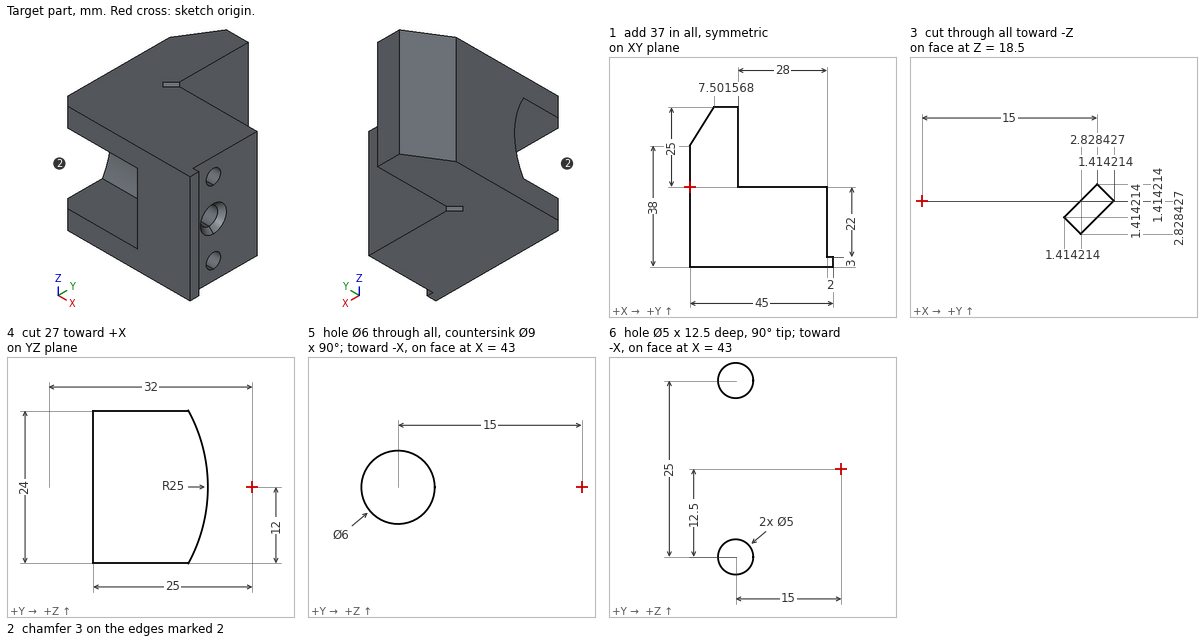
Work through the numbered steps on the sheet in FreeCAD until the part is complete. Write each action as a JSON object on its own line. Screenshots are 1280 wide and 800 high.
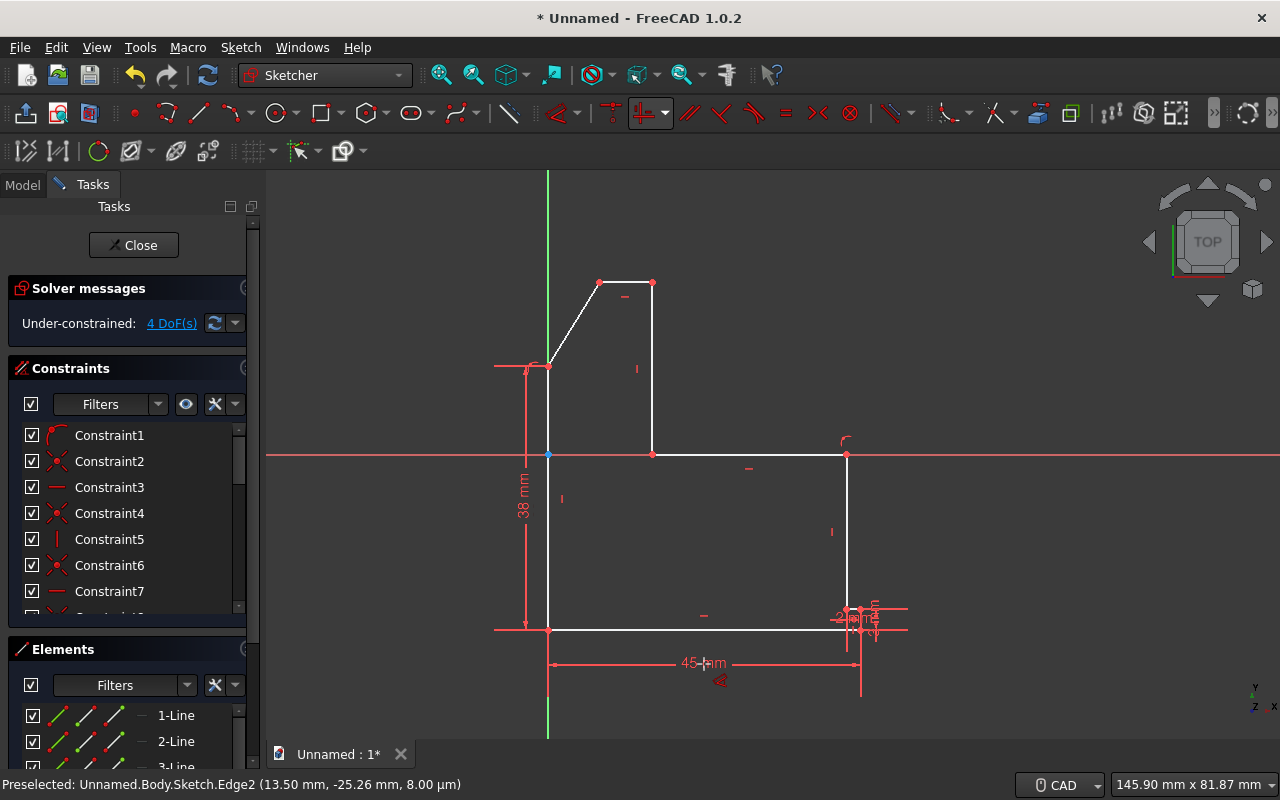
{"action": "left_click", "coordinate": [847, 563]}
{"action": "left_click", "coordinate": [881, 532]}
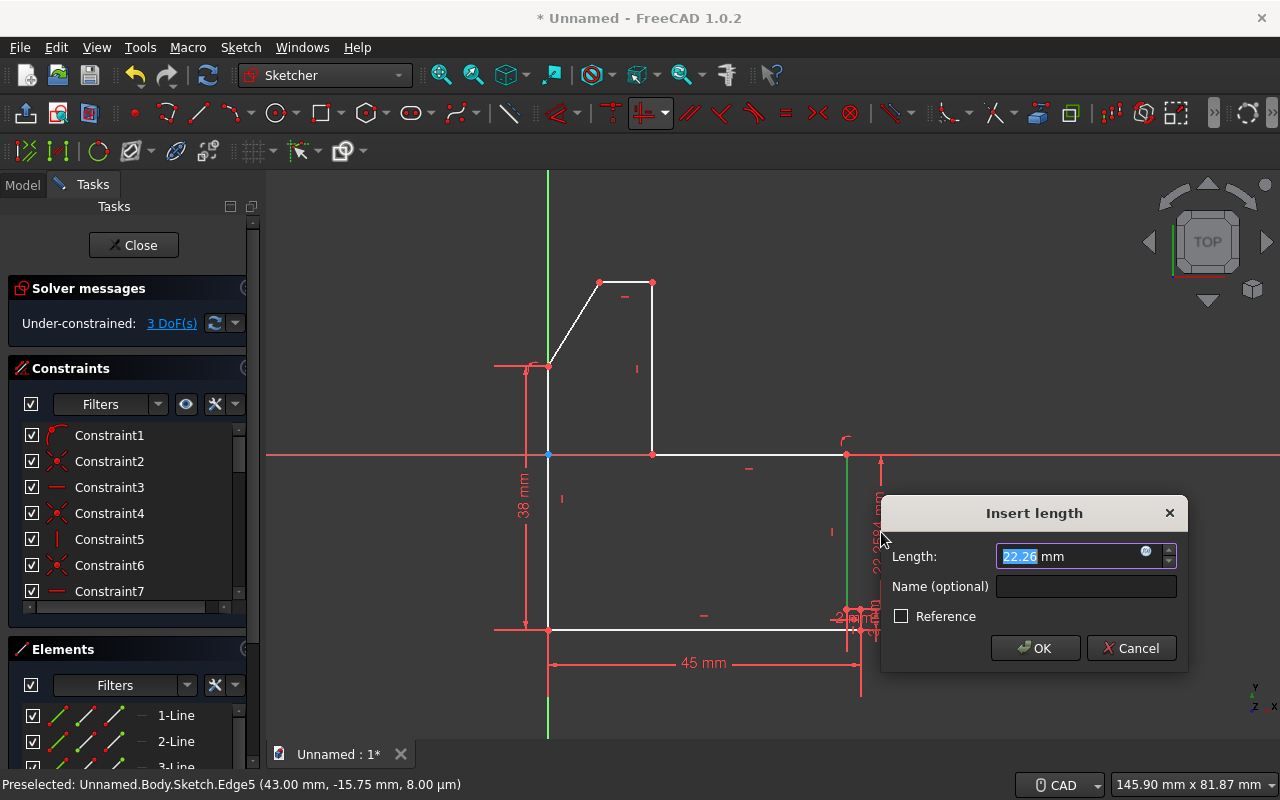
{"action": "type", "text": "22"}
{"action": "key", "text": "Return"}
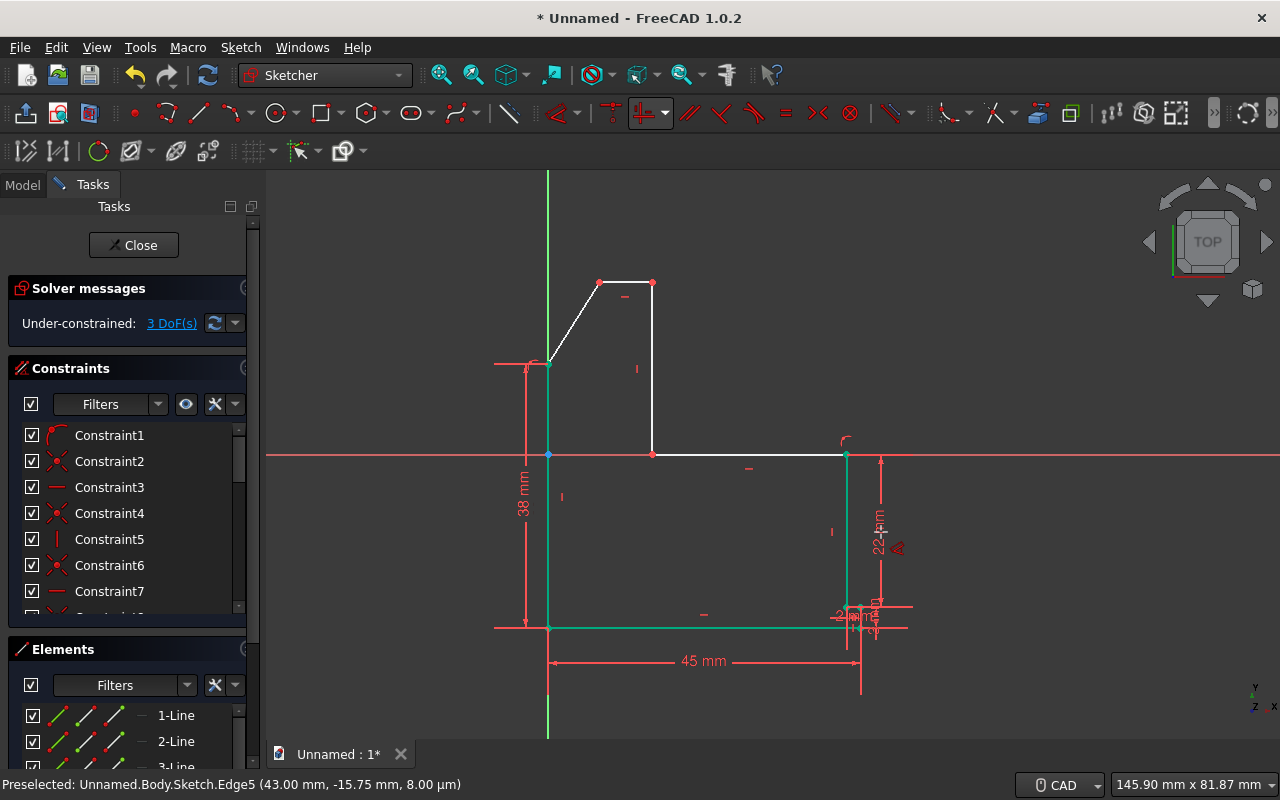
{"action": "left_click", "coordinate": [788, 455]}
{"action": "left_click", "coordinate": [750, 489]}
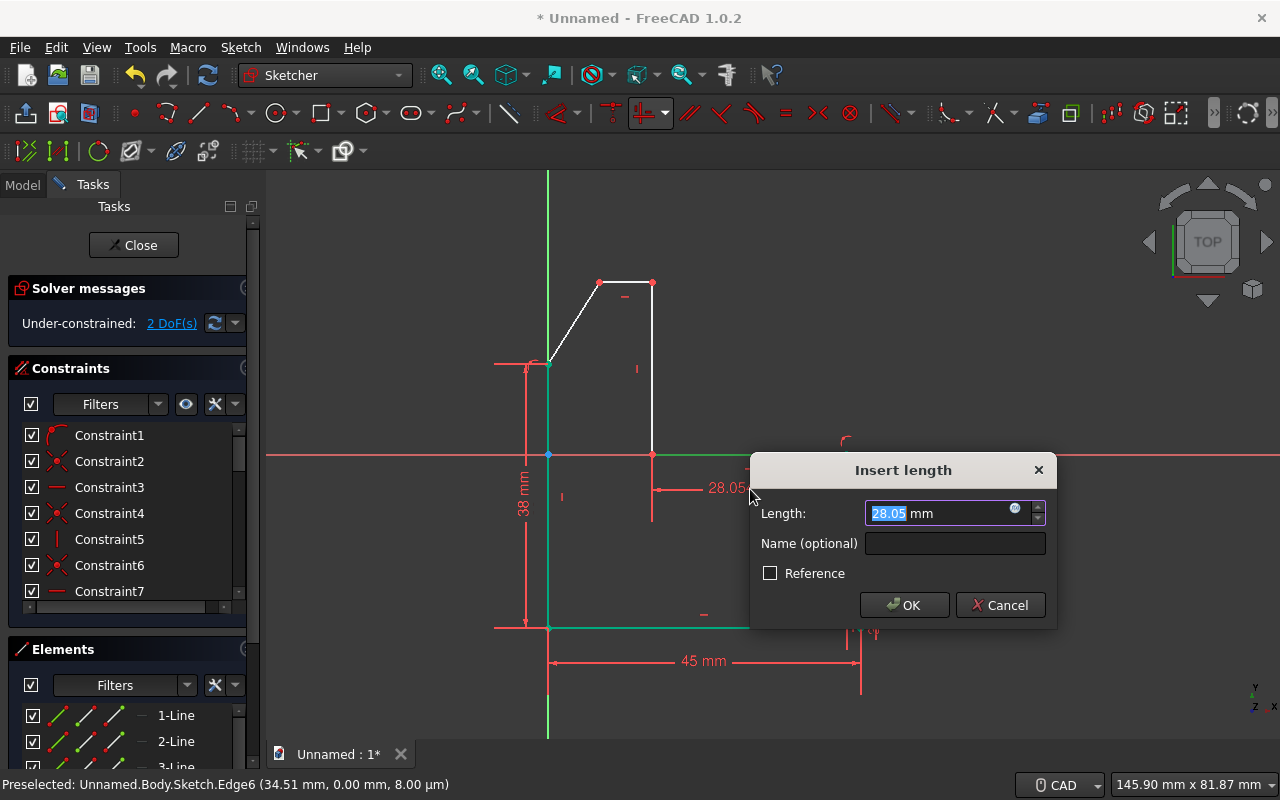
{"action": "type", "text": "28"}
{"action": "key", "text": "Return"}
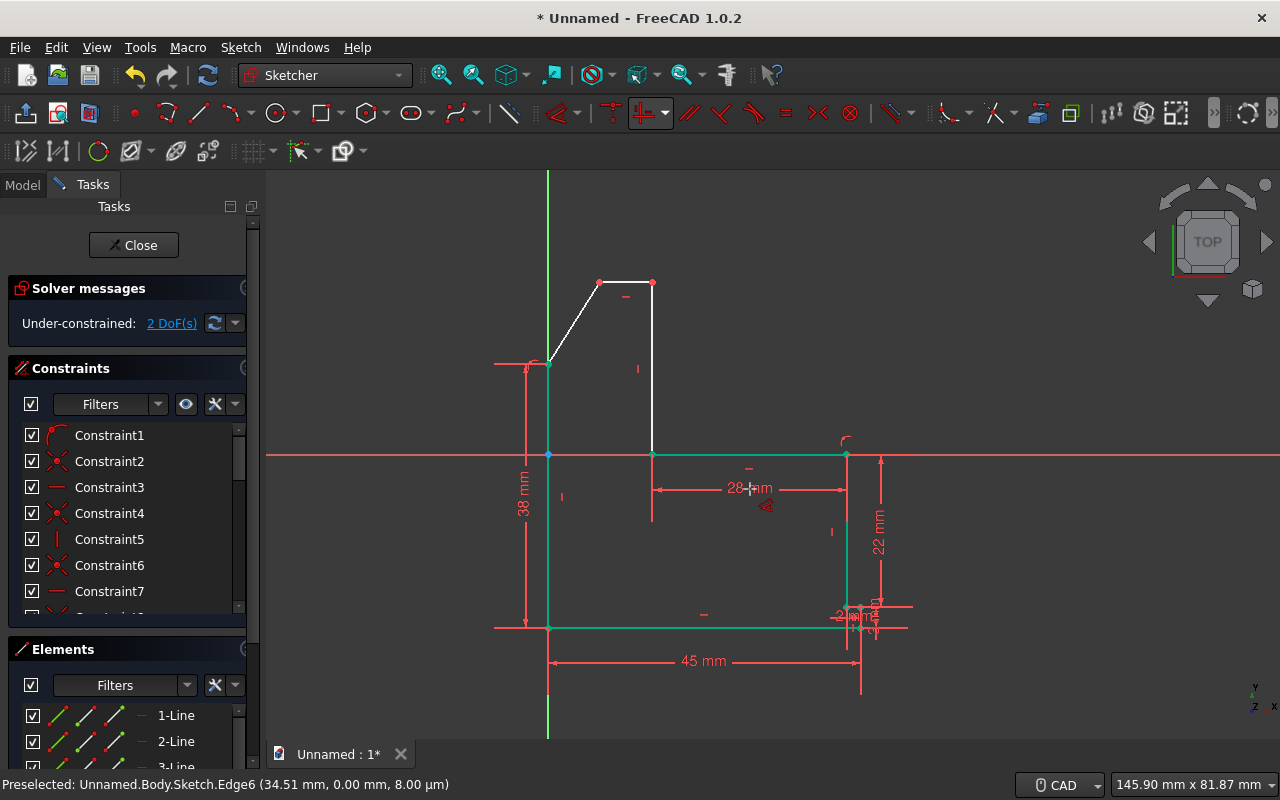
{"action": "left_click", "coordinate": [652, 403]}
{"action": "left_click", "coordinate": [618, 368]}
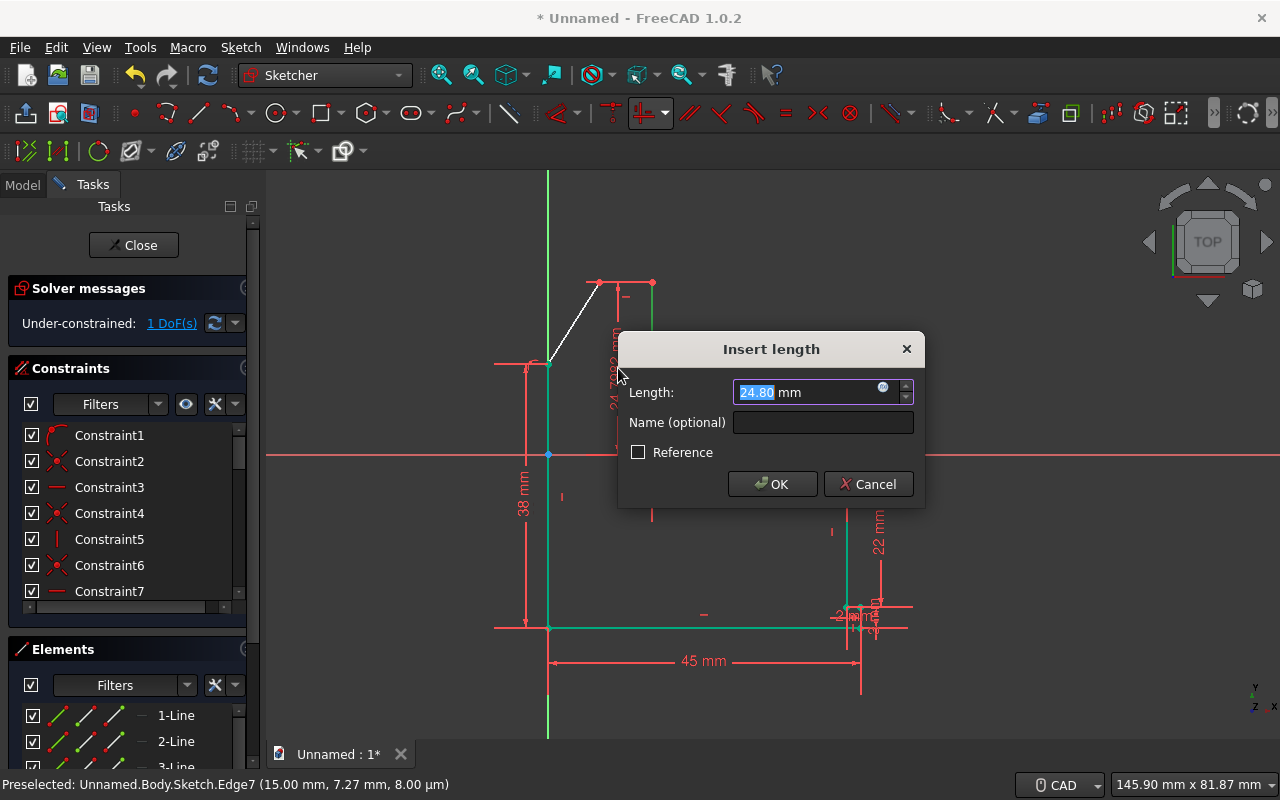
{"action": "type", "text": "25"}
{"action": "key", "text": "Return"}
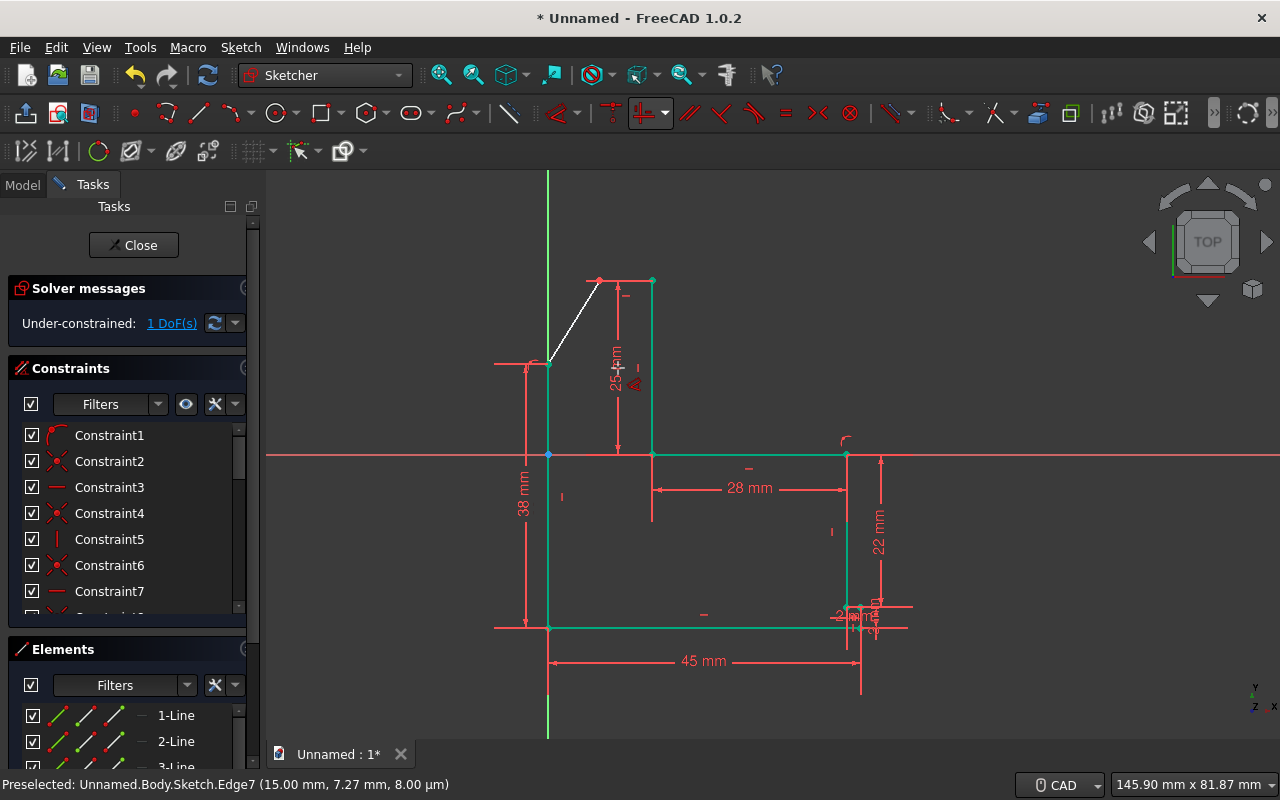
{"action": "left_click", "coordinate": [637, 281]}
{"action": "left_click", "coordinate": [626, 247]}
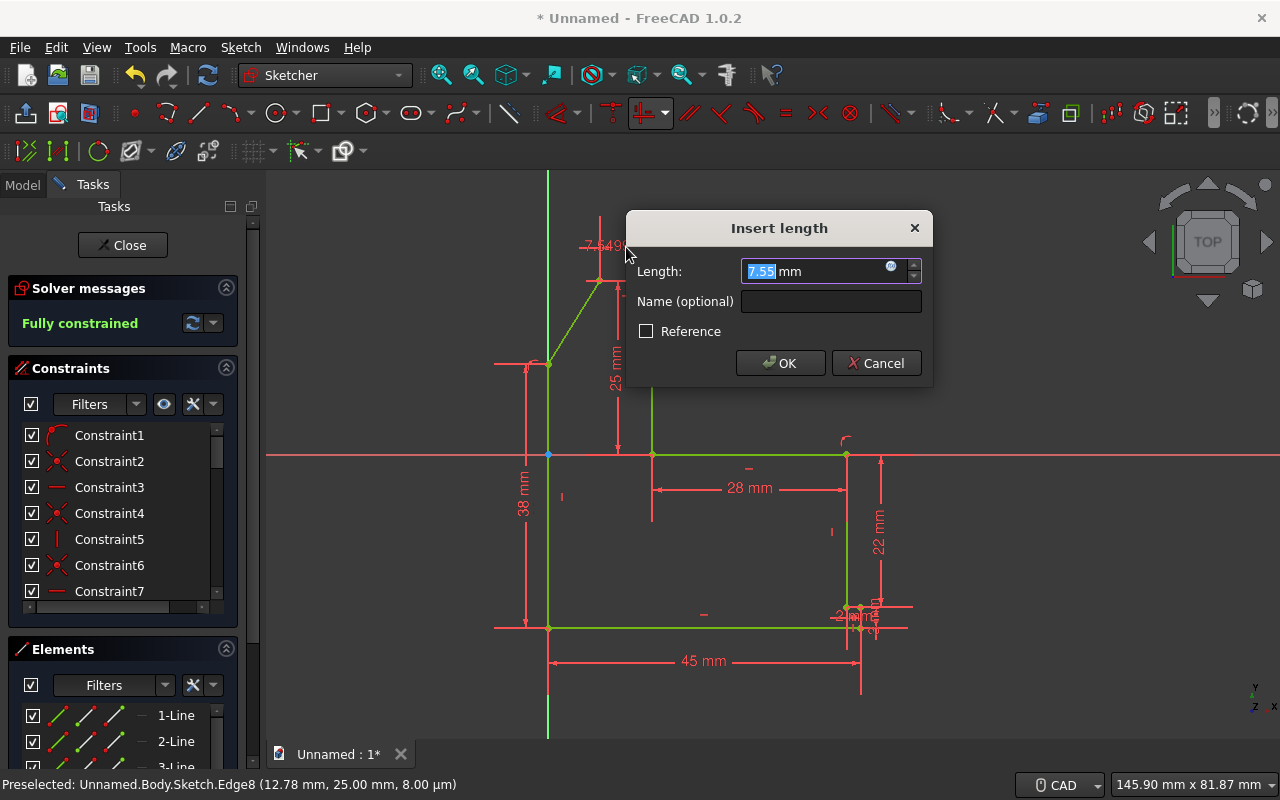
{"action": "type", "text": "7.501568"}
{"action": "key", "text": "Return"}
{"action": "key", "text": "Escape"}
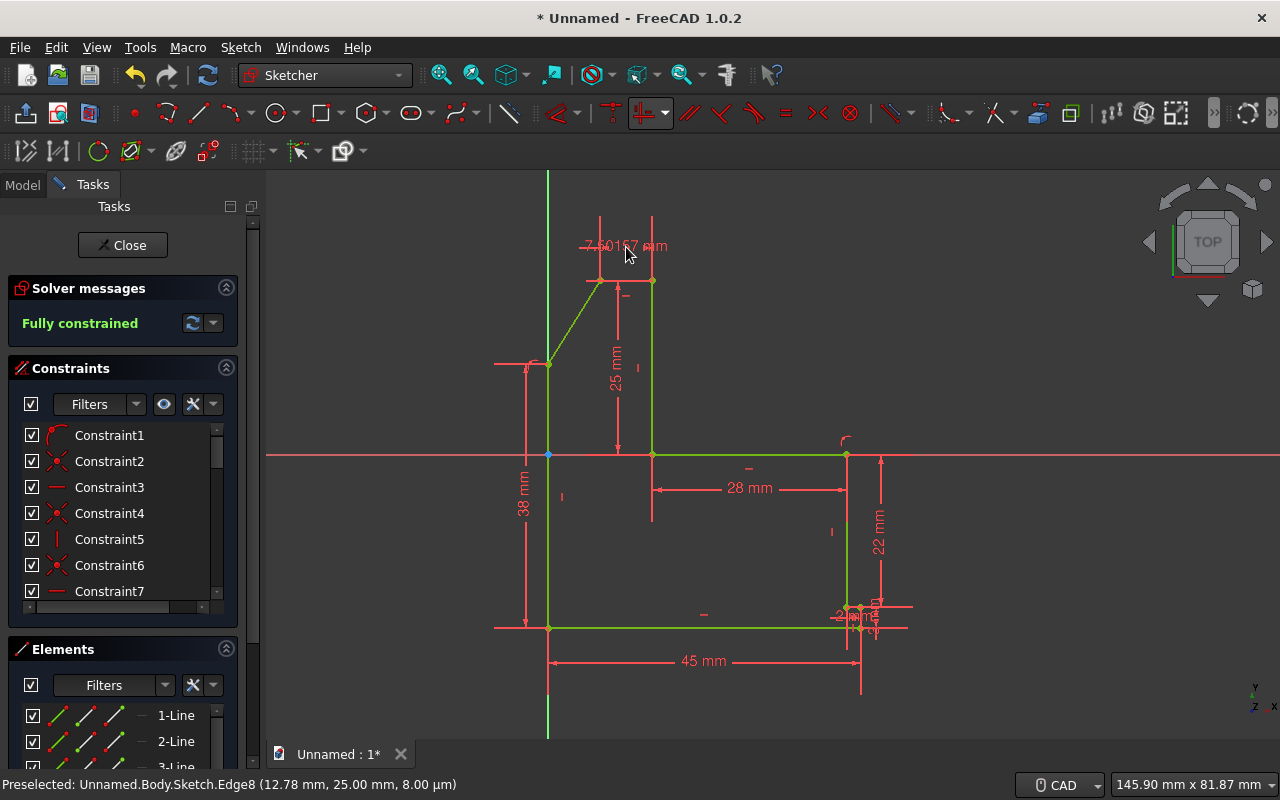
{"action": "left_click", "coordinate": [123, 245]}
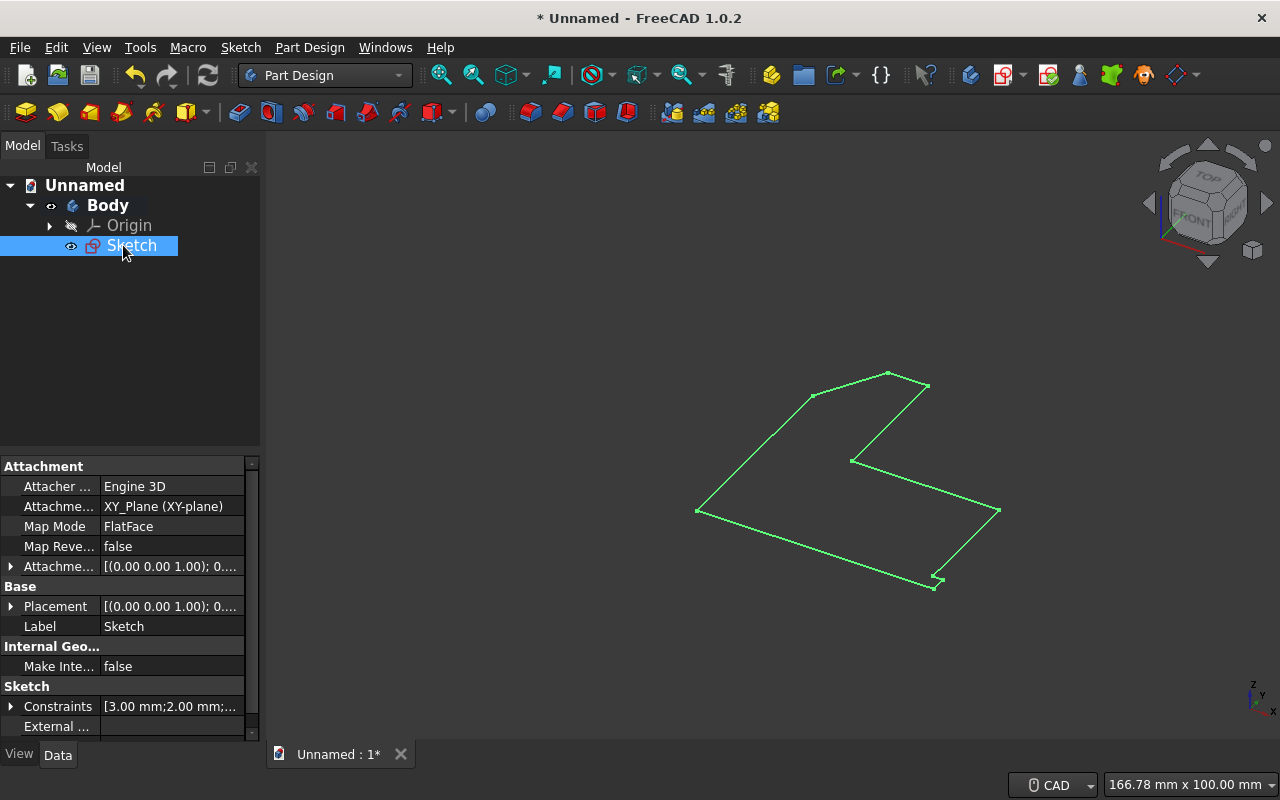
{"action": "left_click", "coordinate": [26, 112]}